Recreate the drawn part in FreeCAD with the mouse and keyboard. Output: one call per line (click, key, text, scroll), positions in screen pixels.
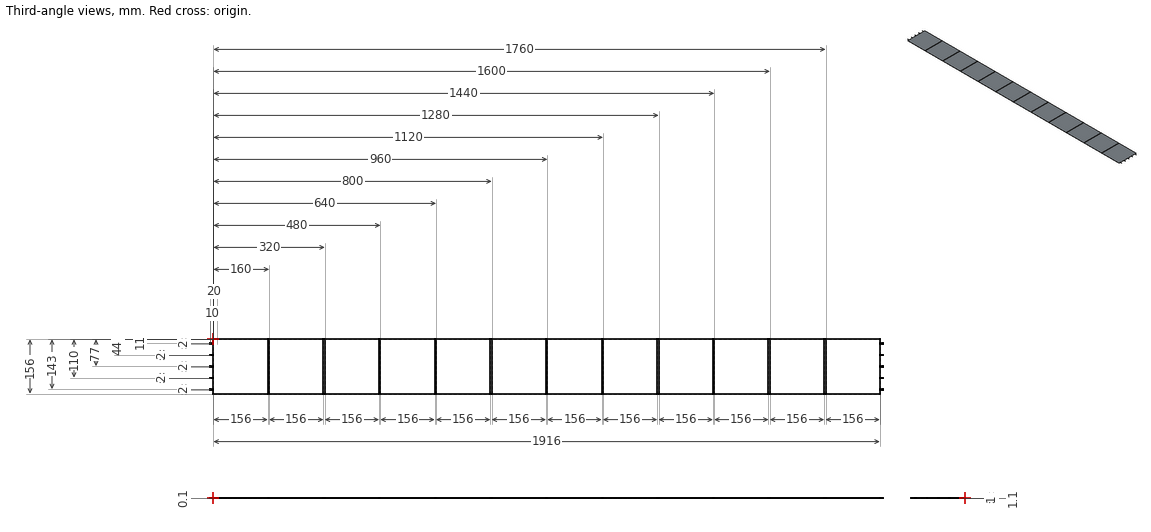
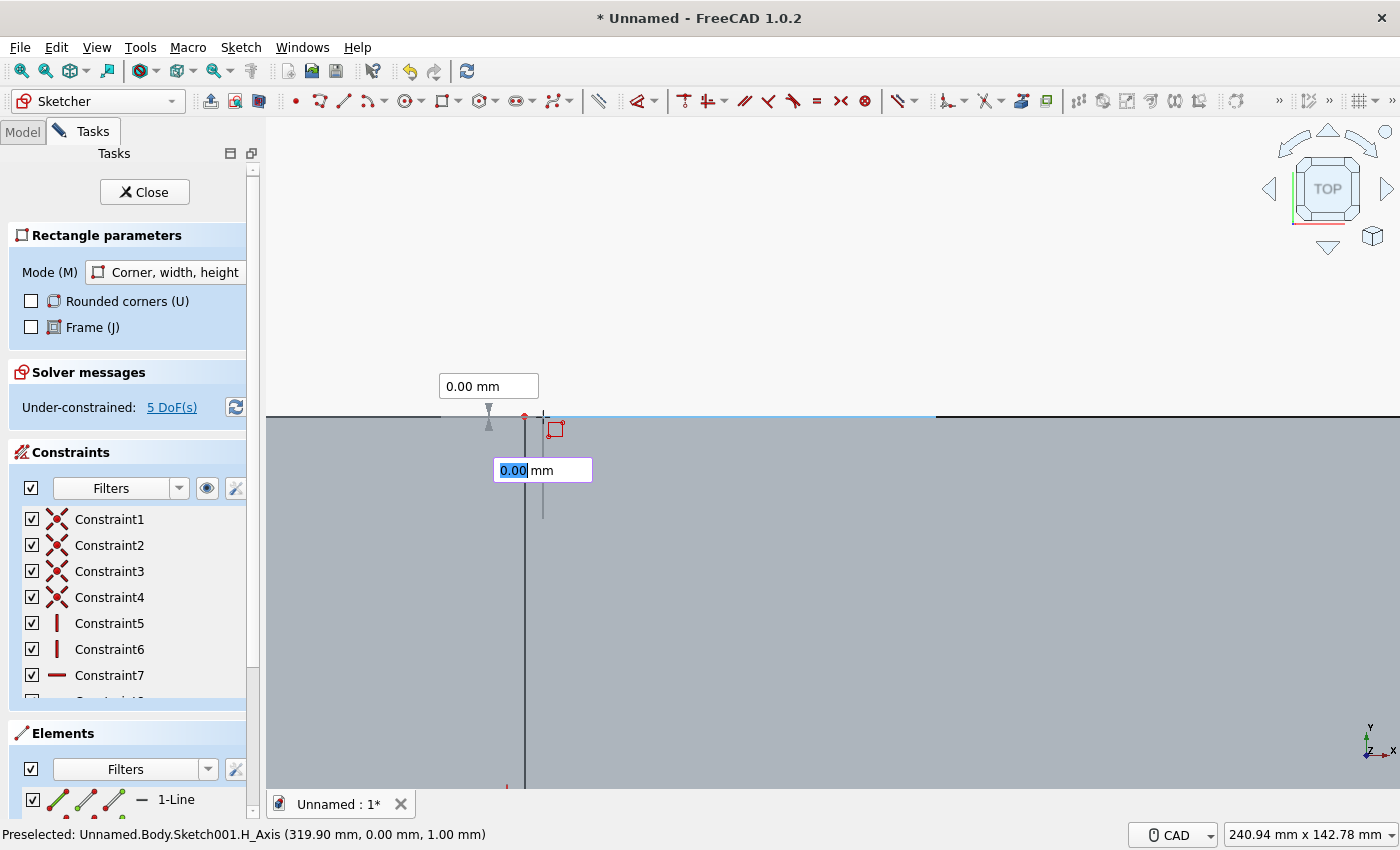
scroll(541, 426, down, 13)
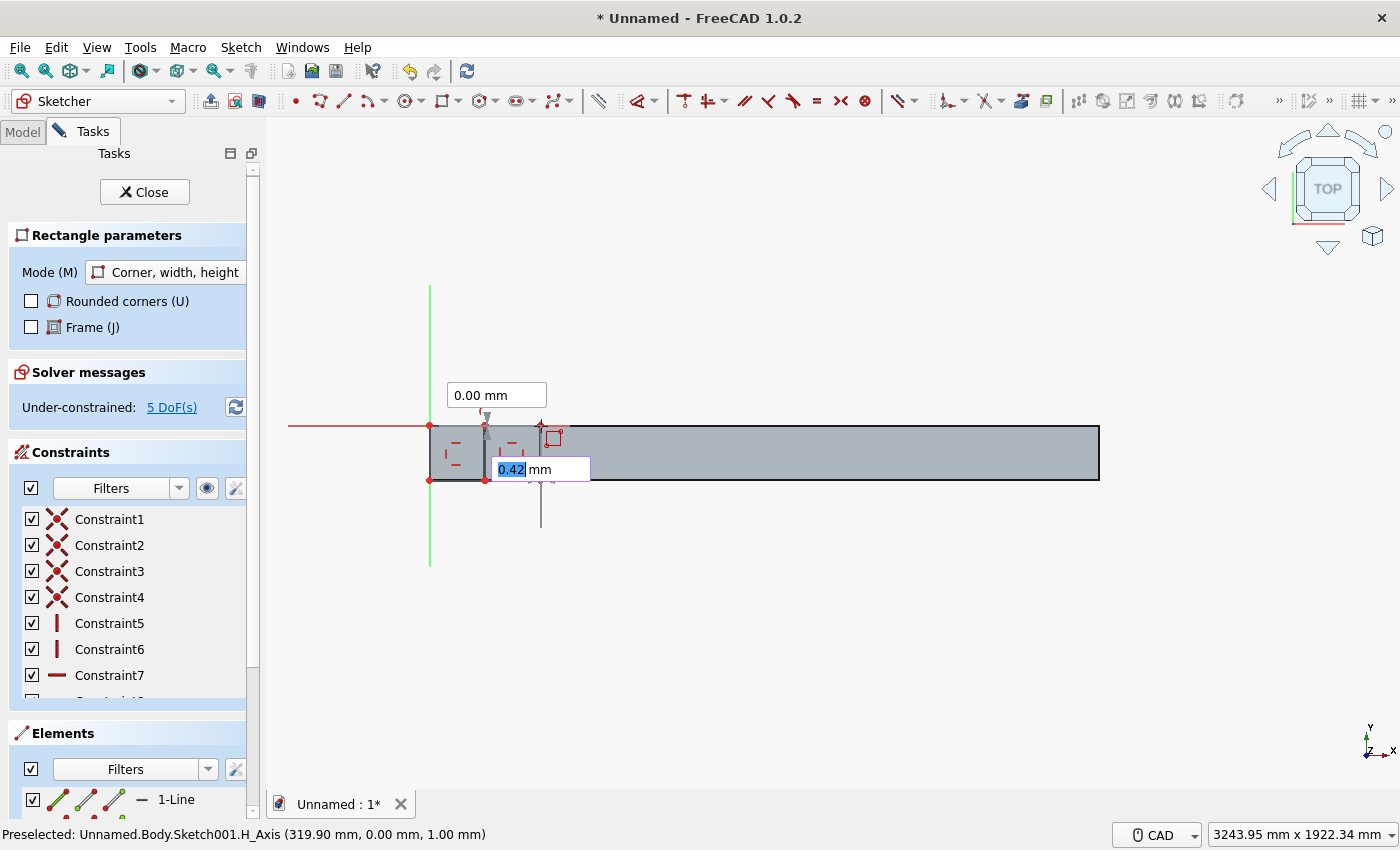
click(596, 480)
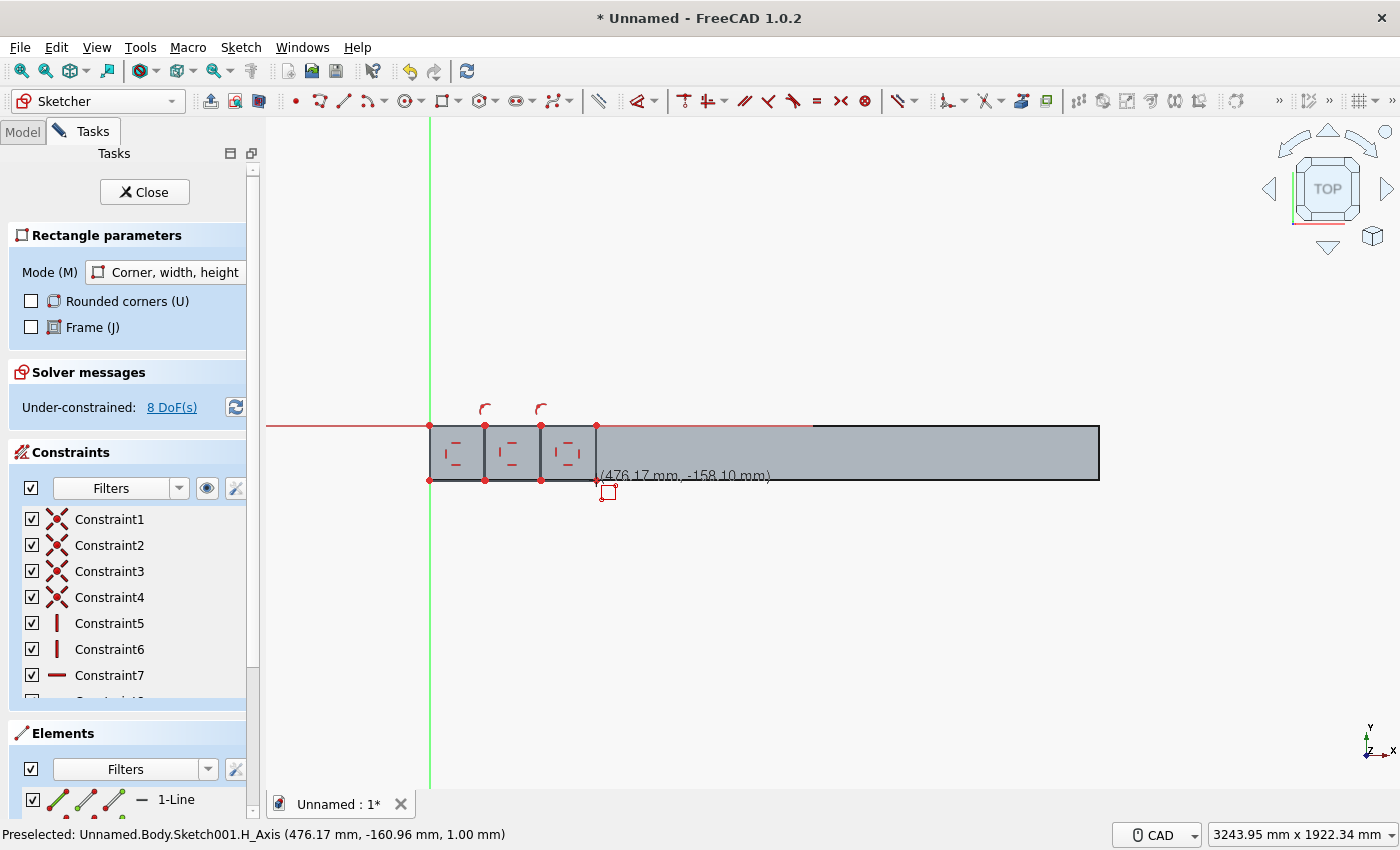
scroll(597, 426, up, 13)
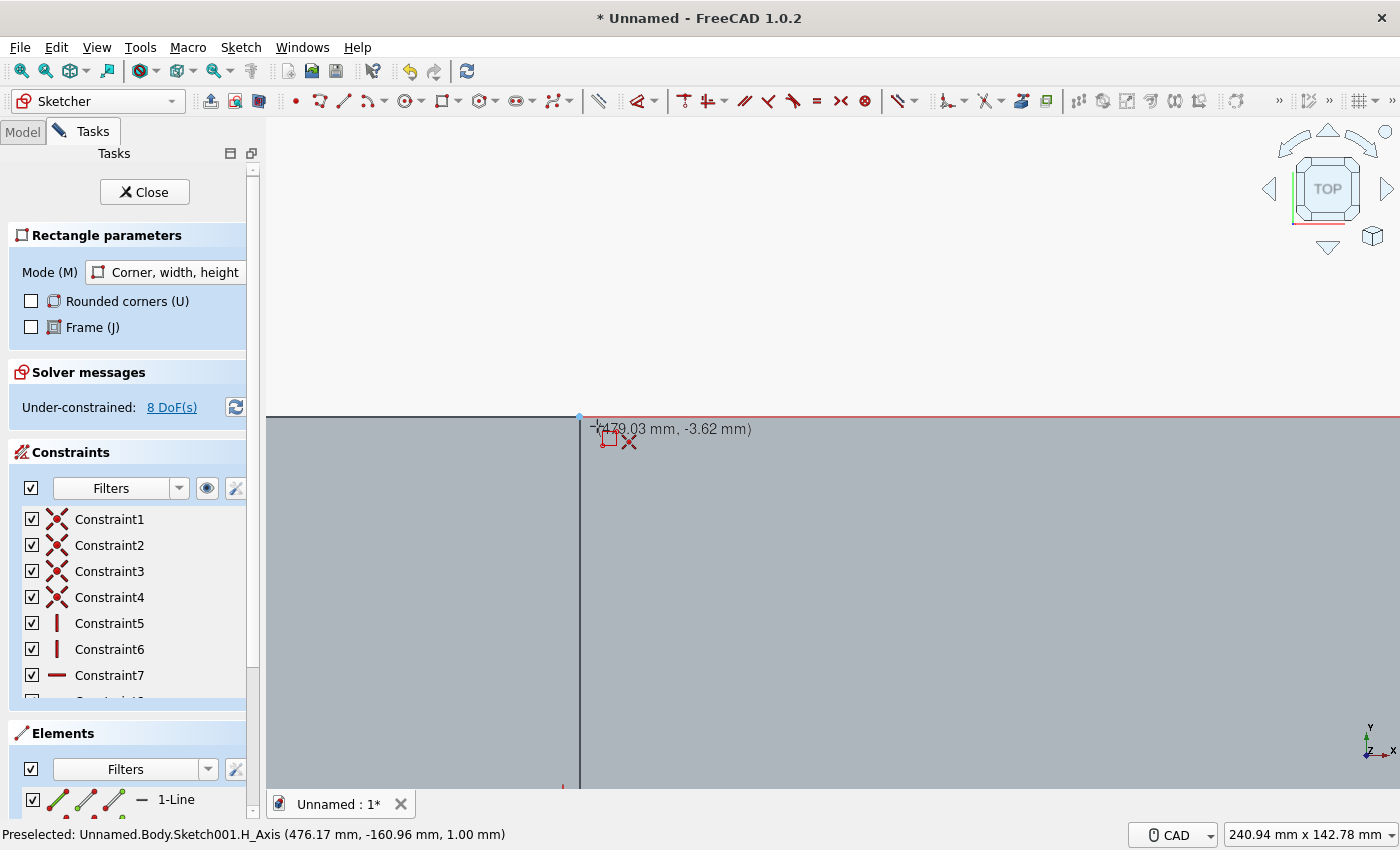
click(598, 417)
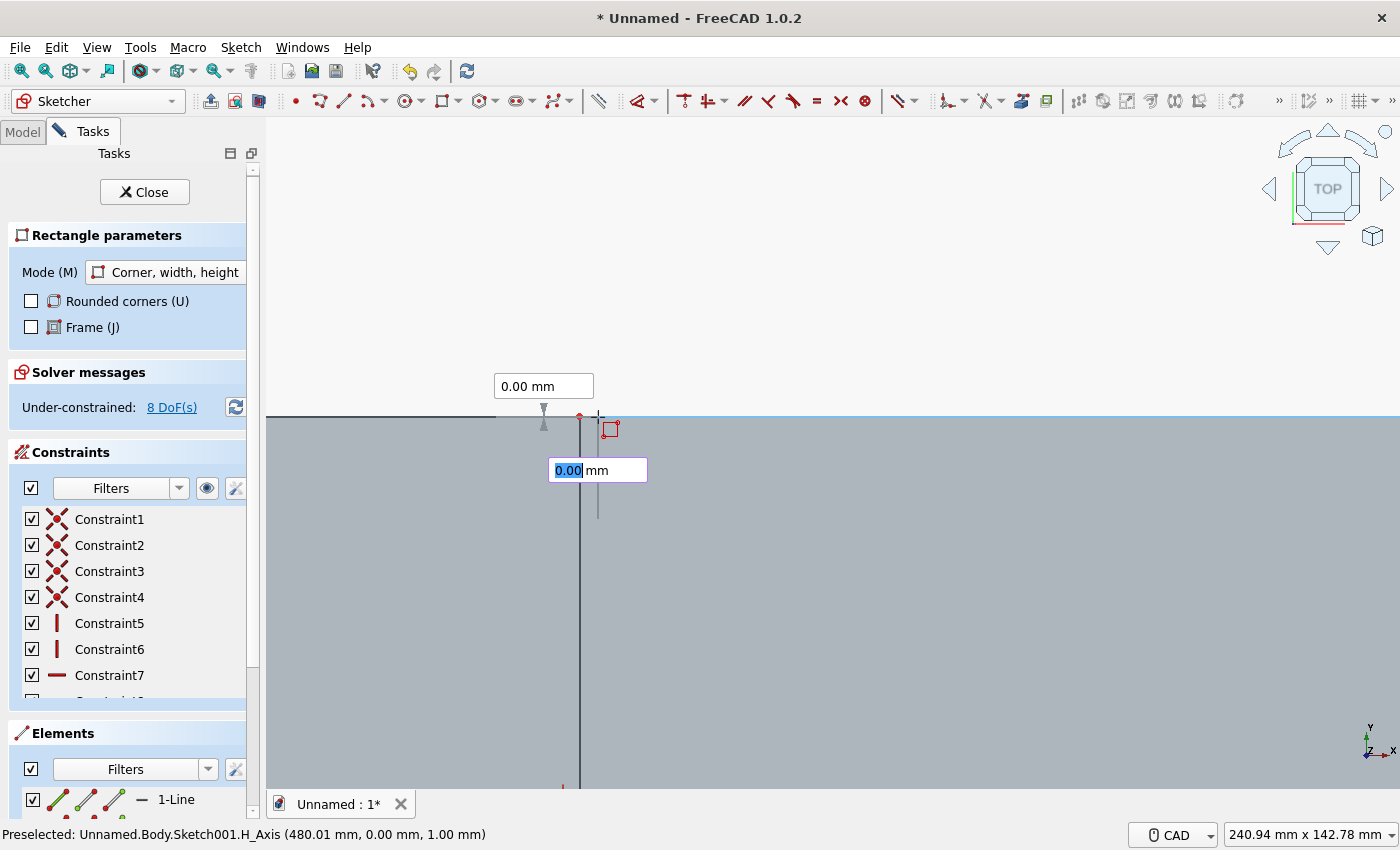
scroll(597, 426, down, 13)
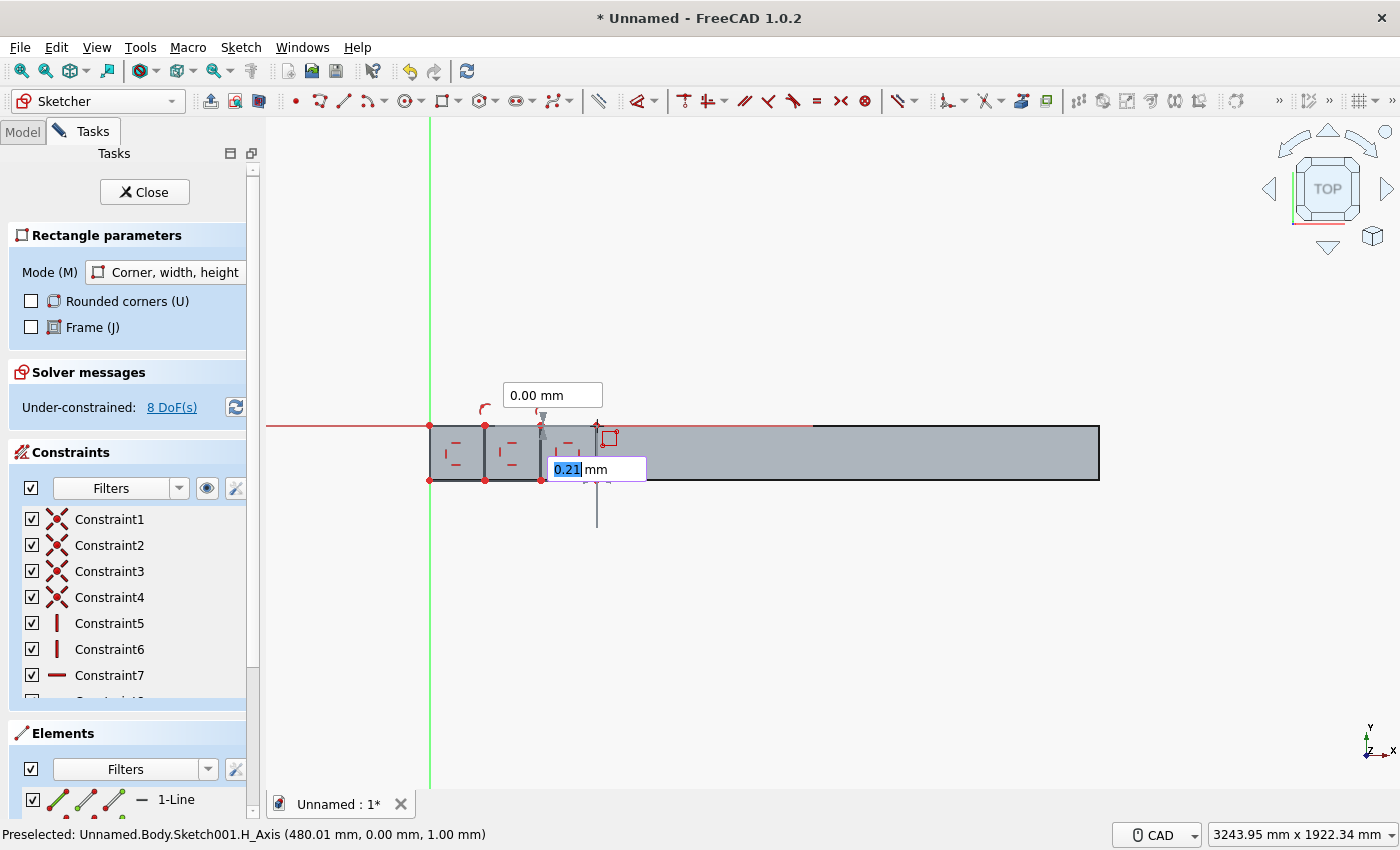
click(652, 480)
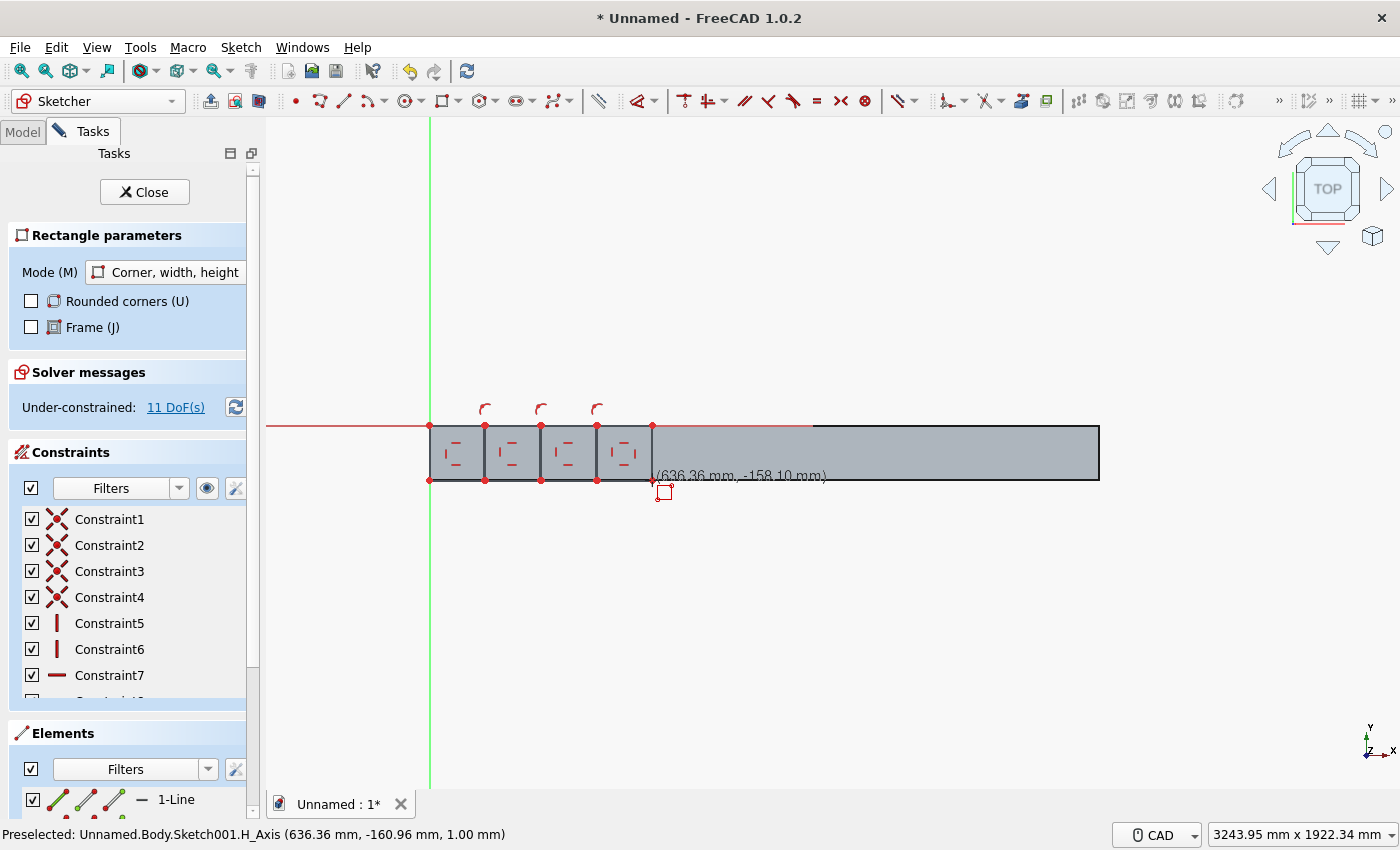
scroll(653, 426, up, 13)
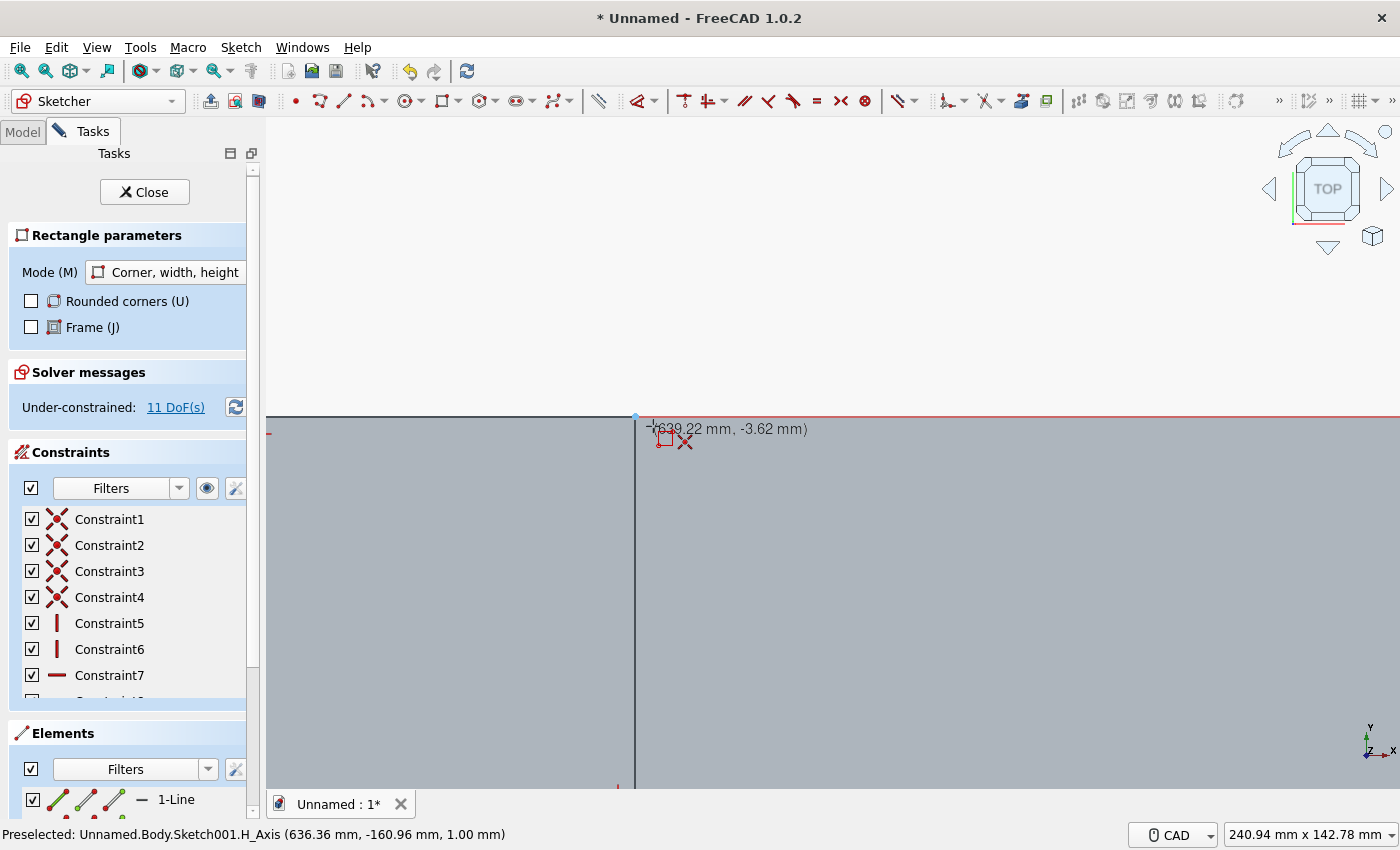
click(652, 417)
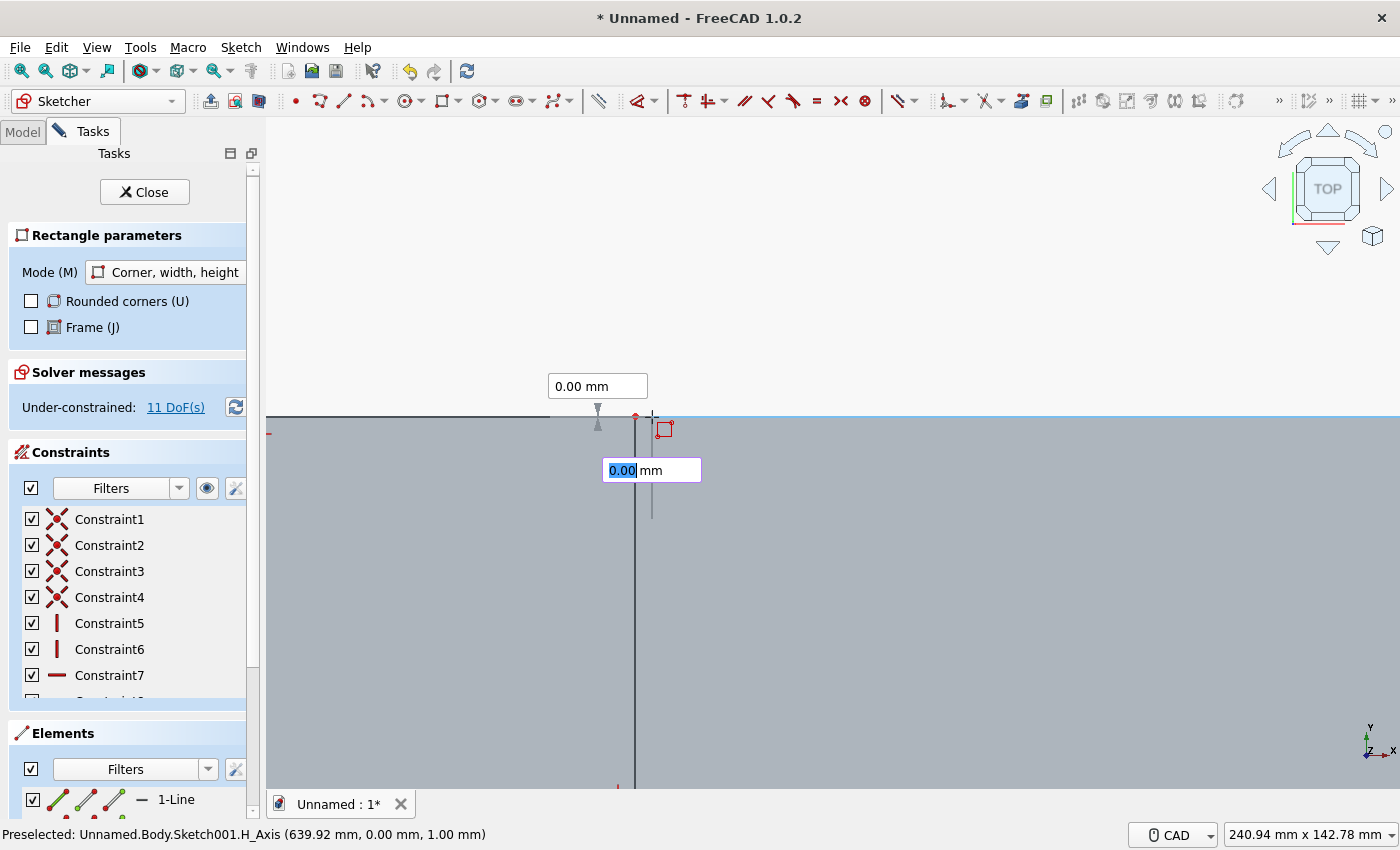
scroll(653, 426, down, 13)